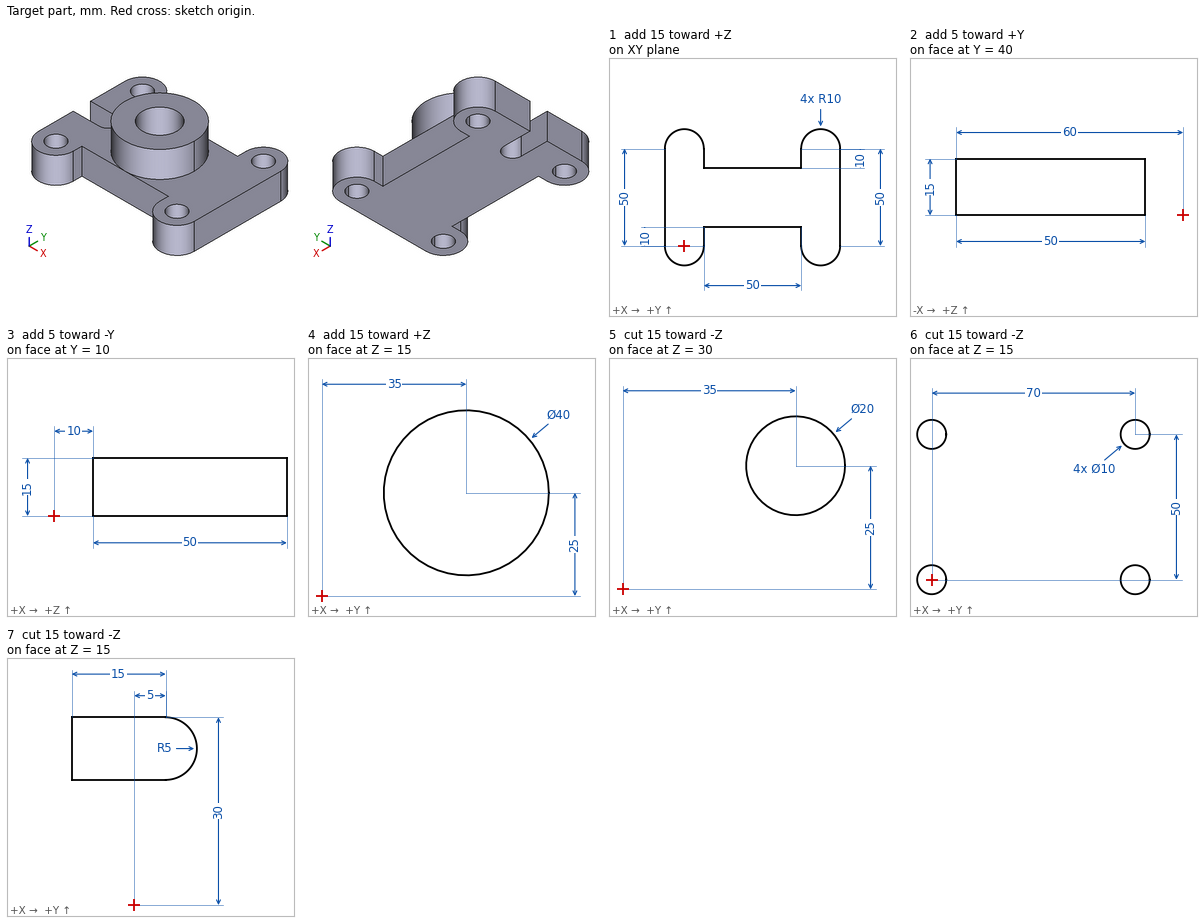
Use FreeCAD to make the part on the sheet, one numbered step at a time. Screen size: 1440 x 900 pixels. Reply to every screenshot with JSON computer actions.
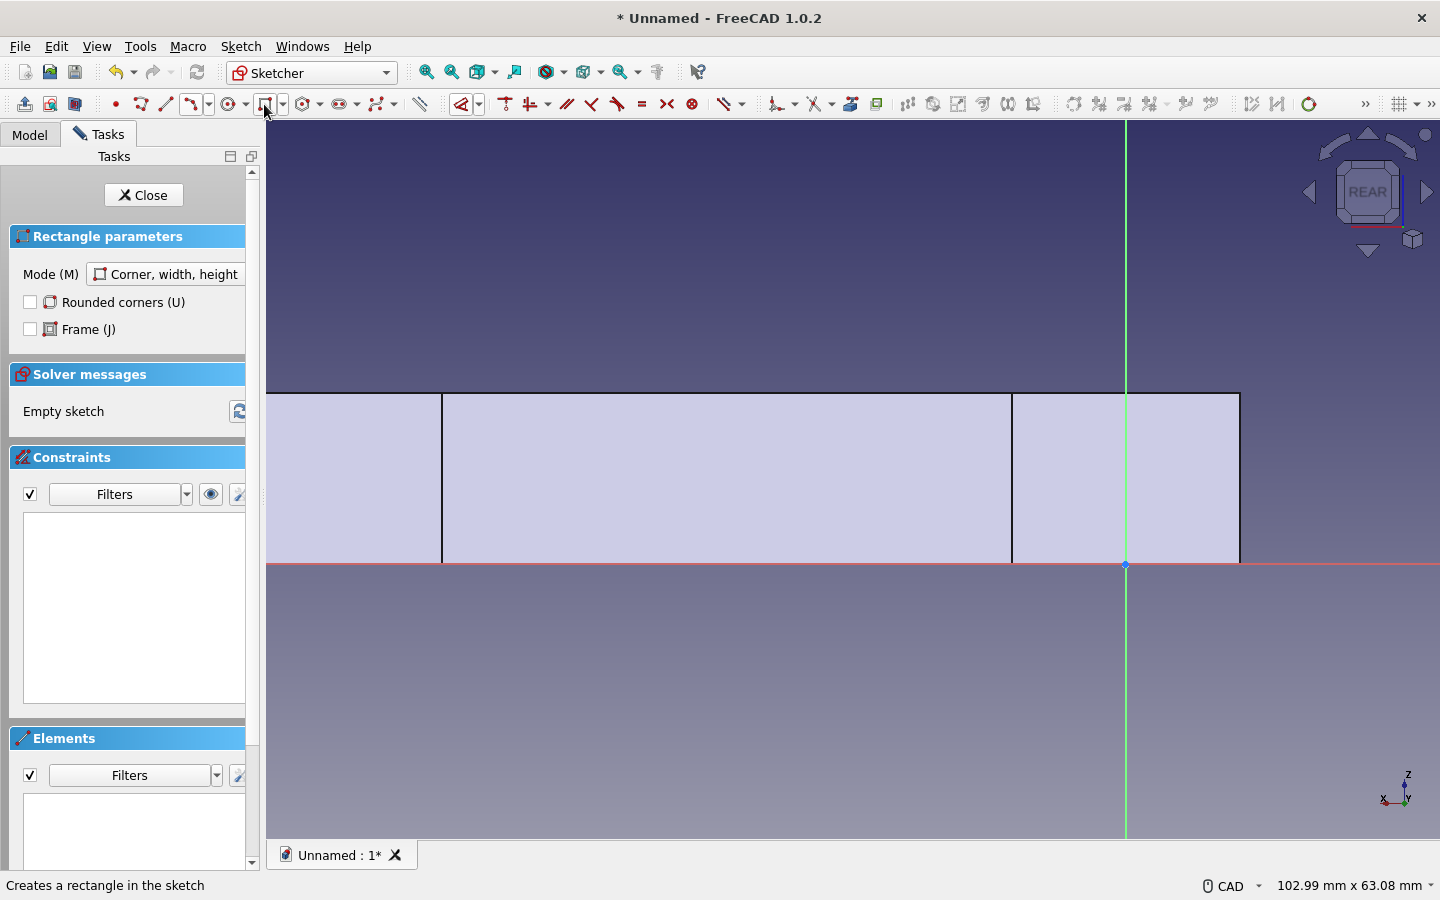
{"action": "left_click", "coordinate": [442, 393]}
{"action": "left_click", "coordinate": [1012, 564]}
{"action": "key", "text": "Escape"}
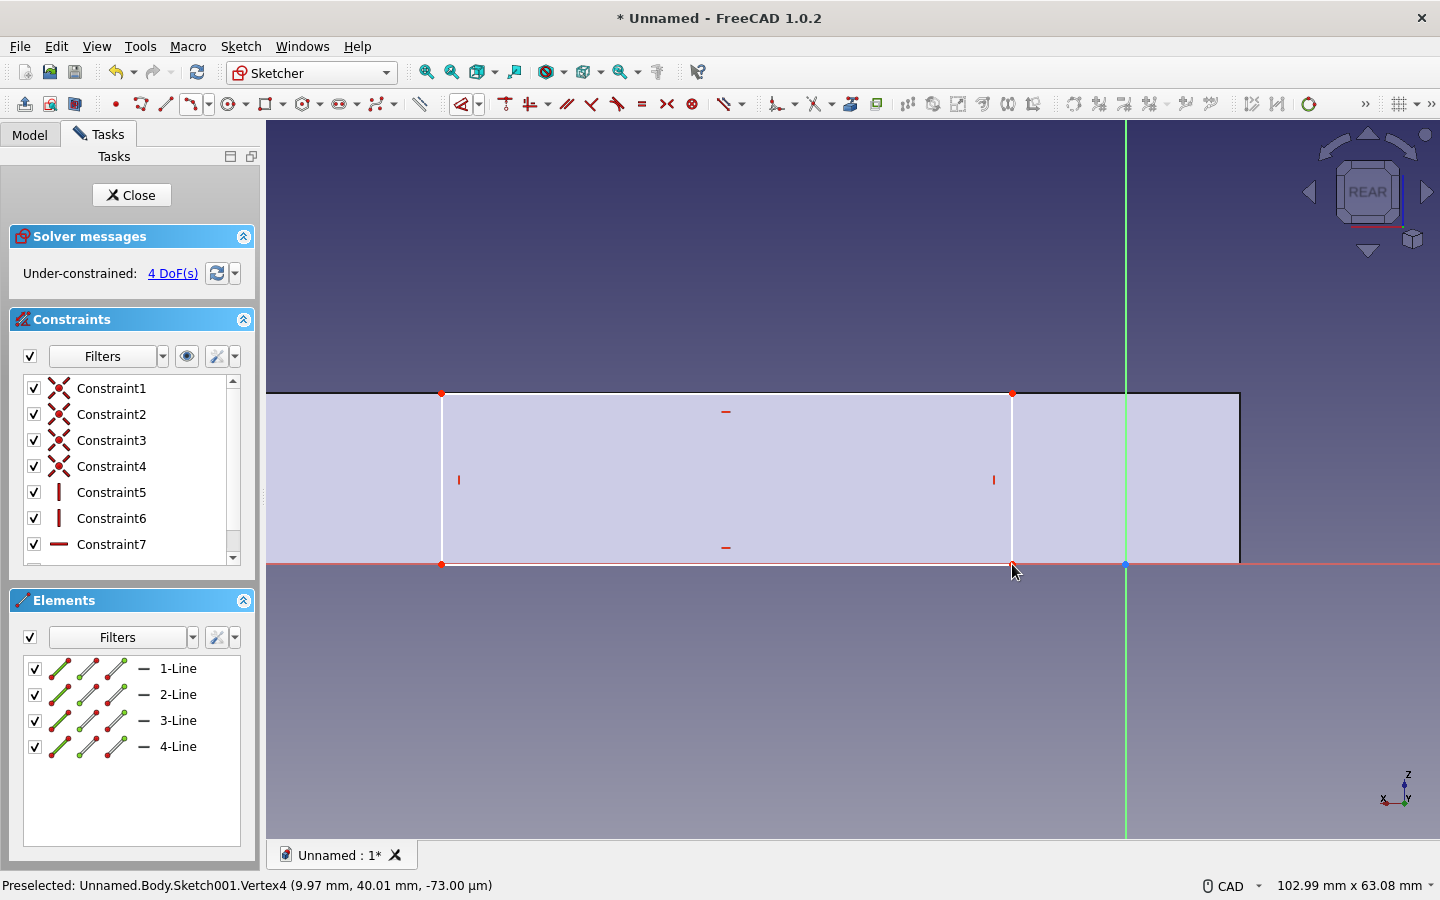
{"action": "left_click", "coordinate": [442, 565]}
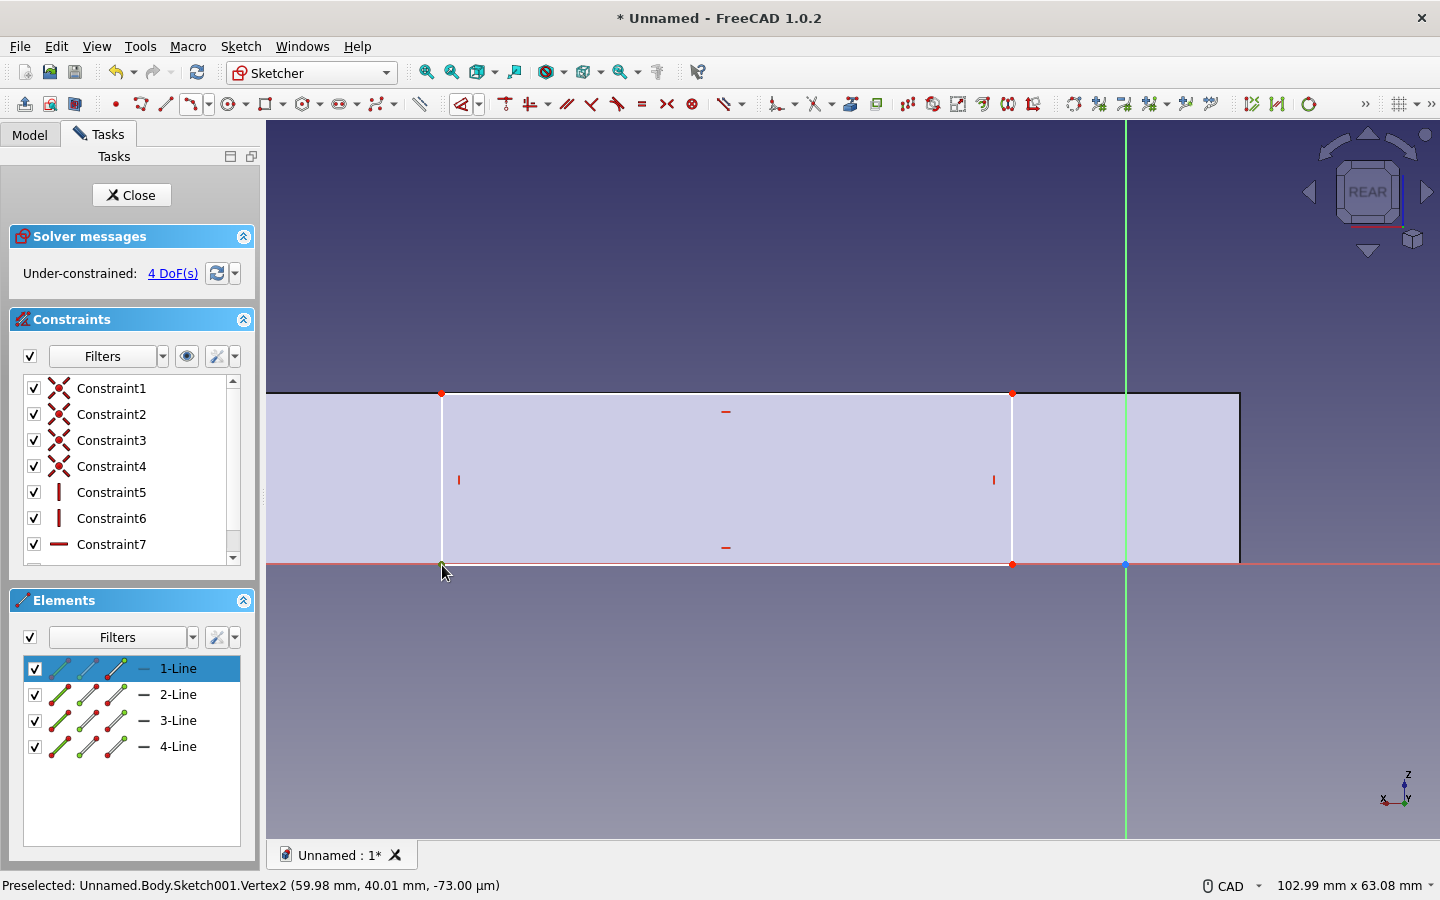
{"action": "left_click", "coordinate": [364, 564]}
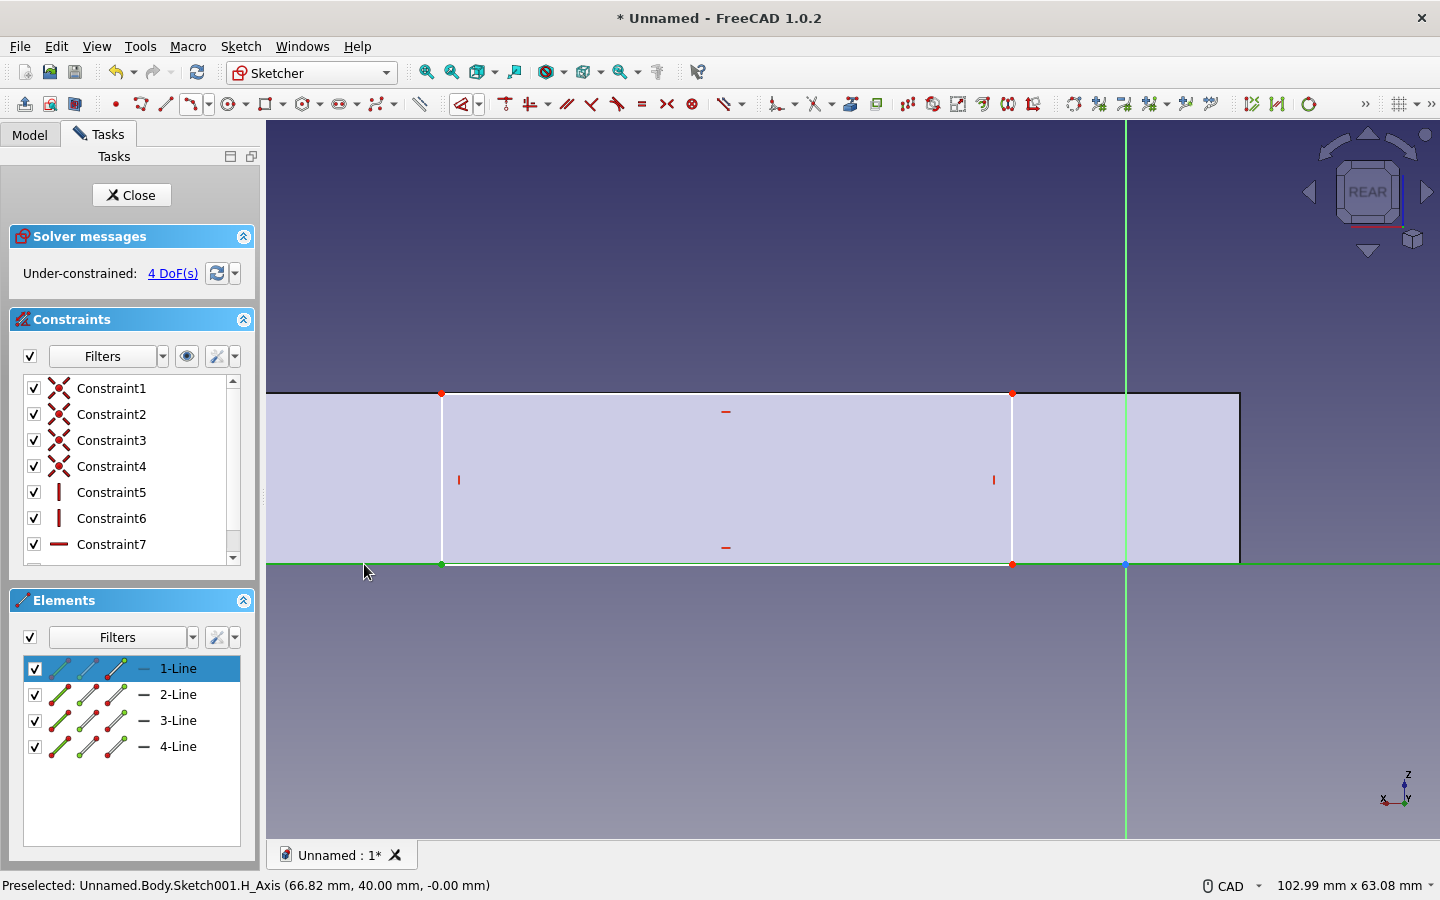
{"action": "left_click", "coordinate": [505, 104]}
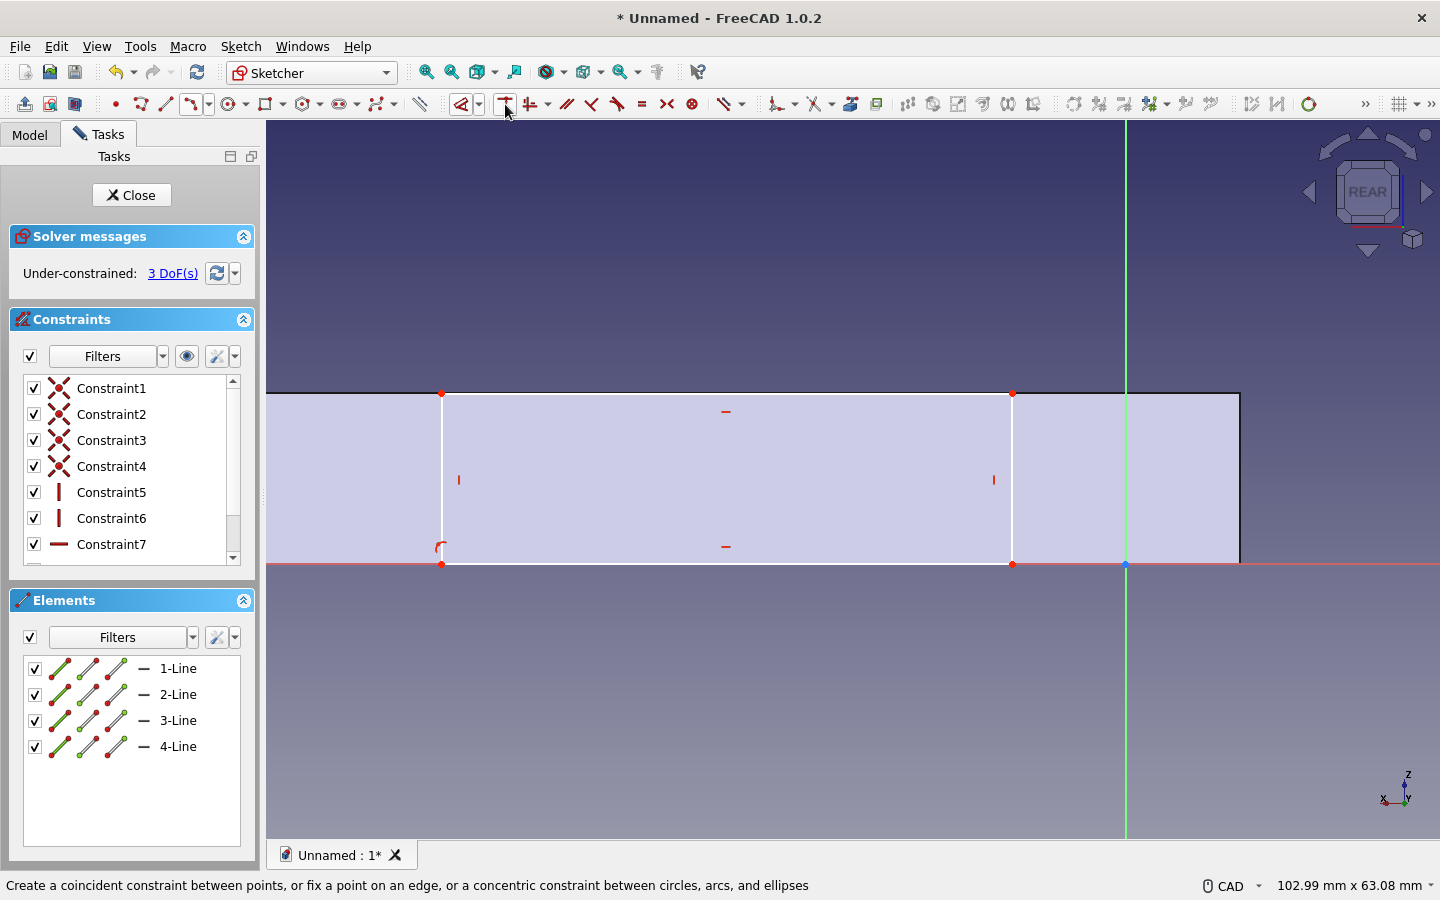
{"action": "left_click", "coordinate": [442, 445]}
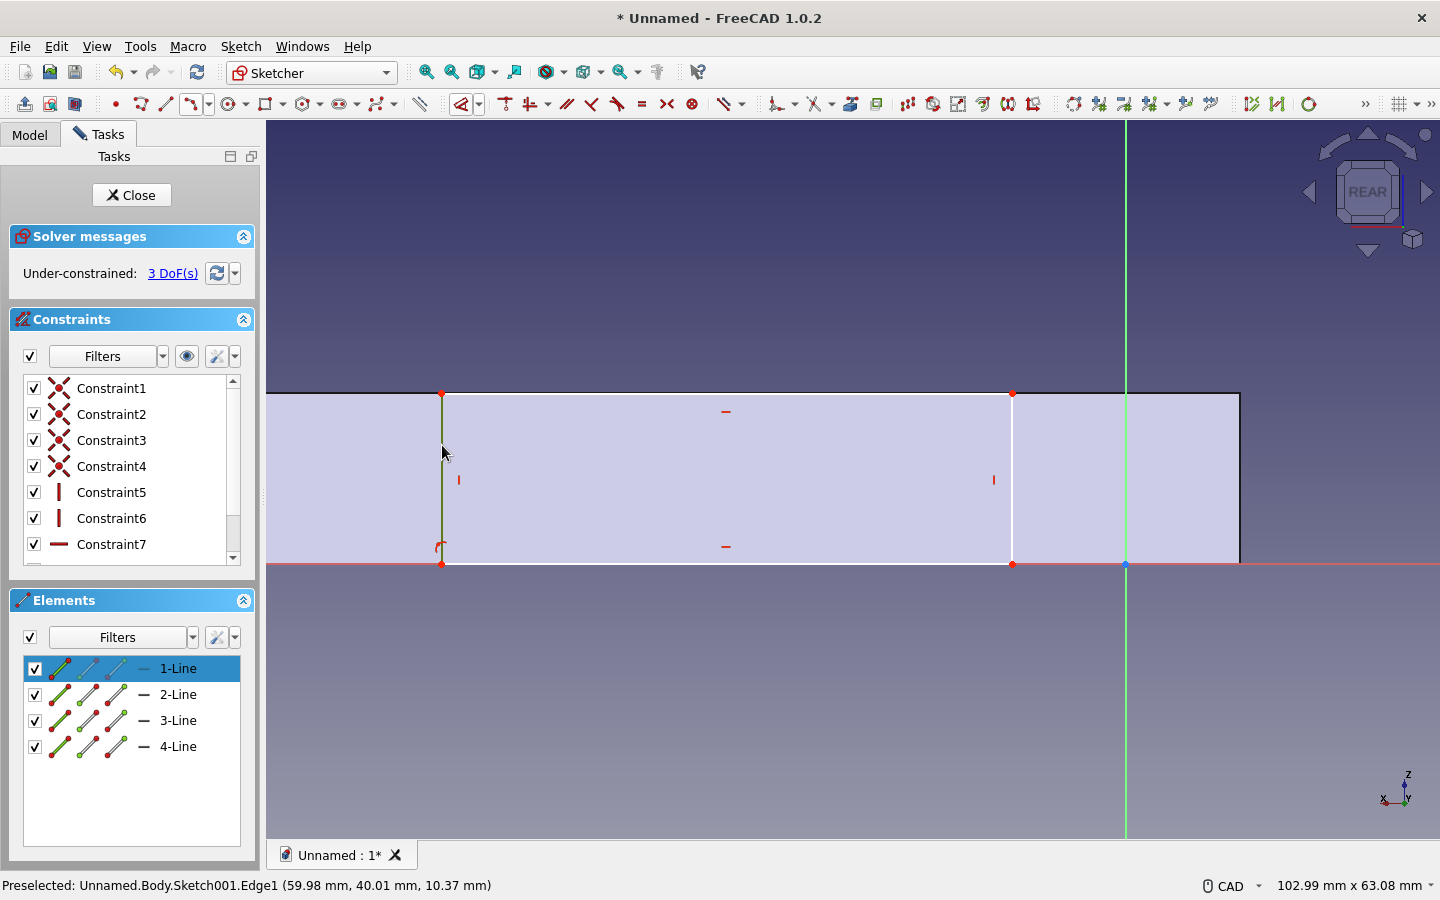
{"action": "left_click", "coordinate": [478, 104]}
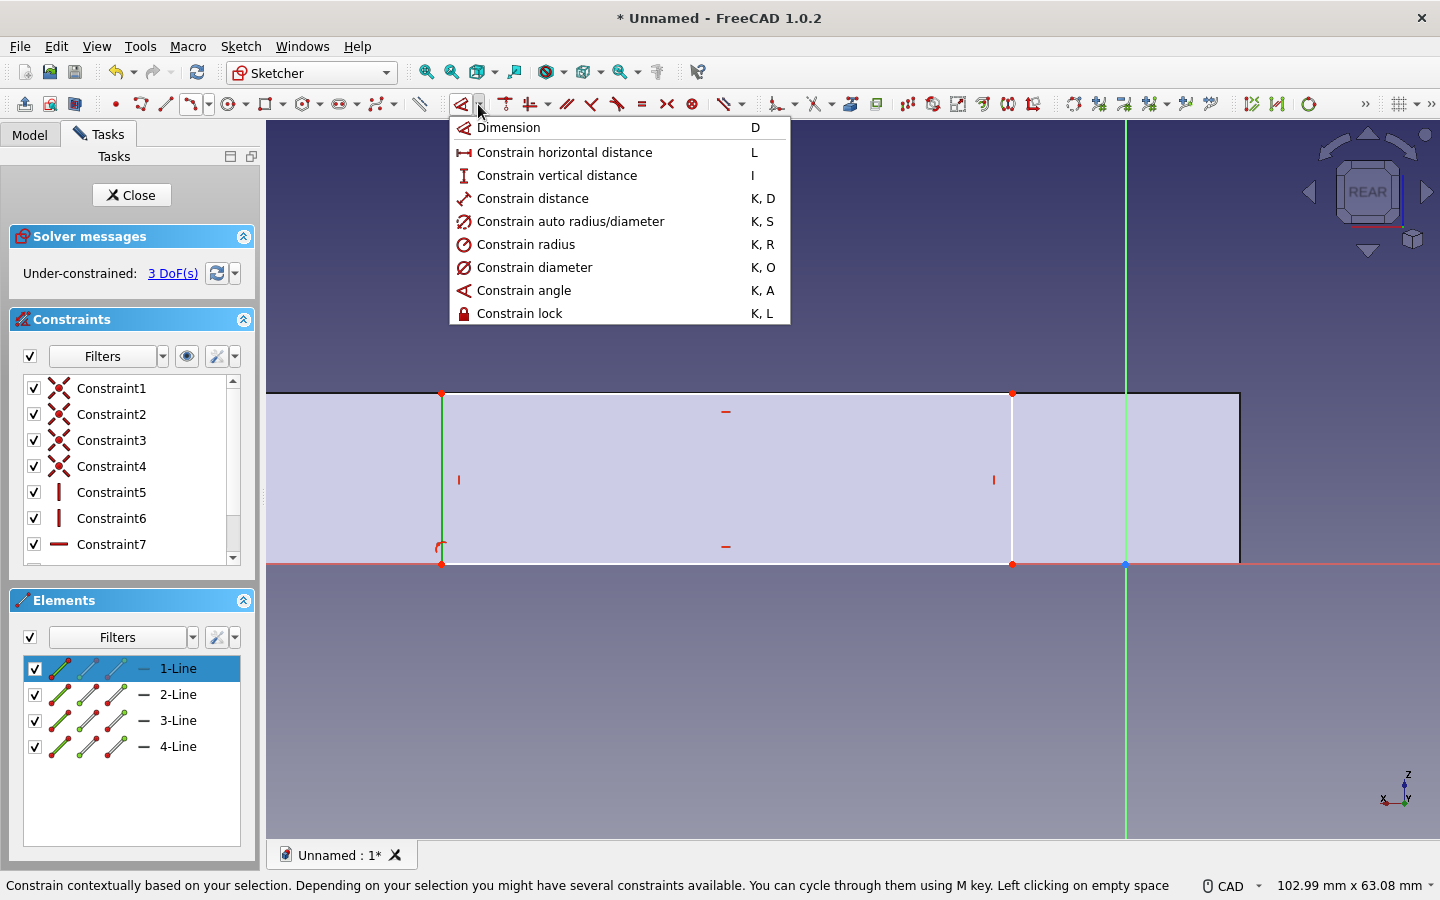
{"action": "left_click", "coordinate": [620, 176]}